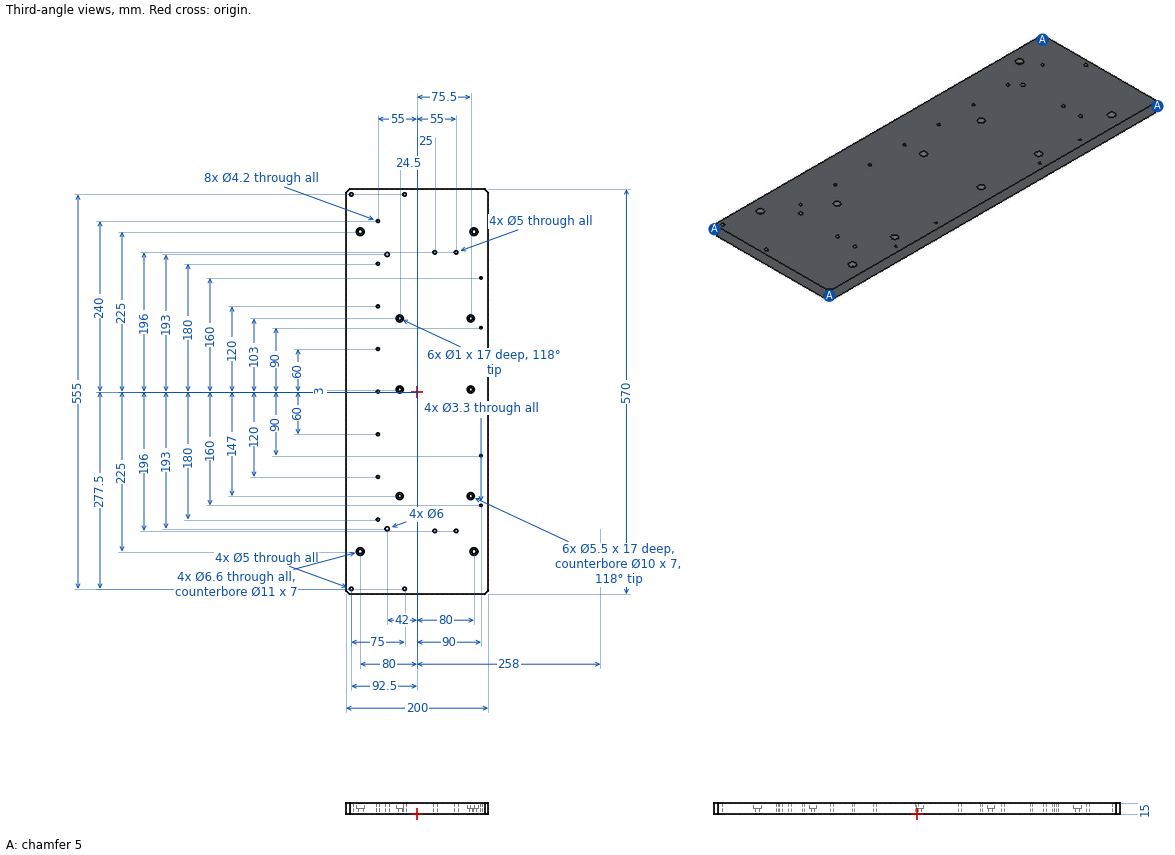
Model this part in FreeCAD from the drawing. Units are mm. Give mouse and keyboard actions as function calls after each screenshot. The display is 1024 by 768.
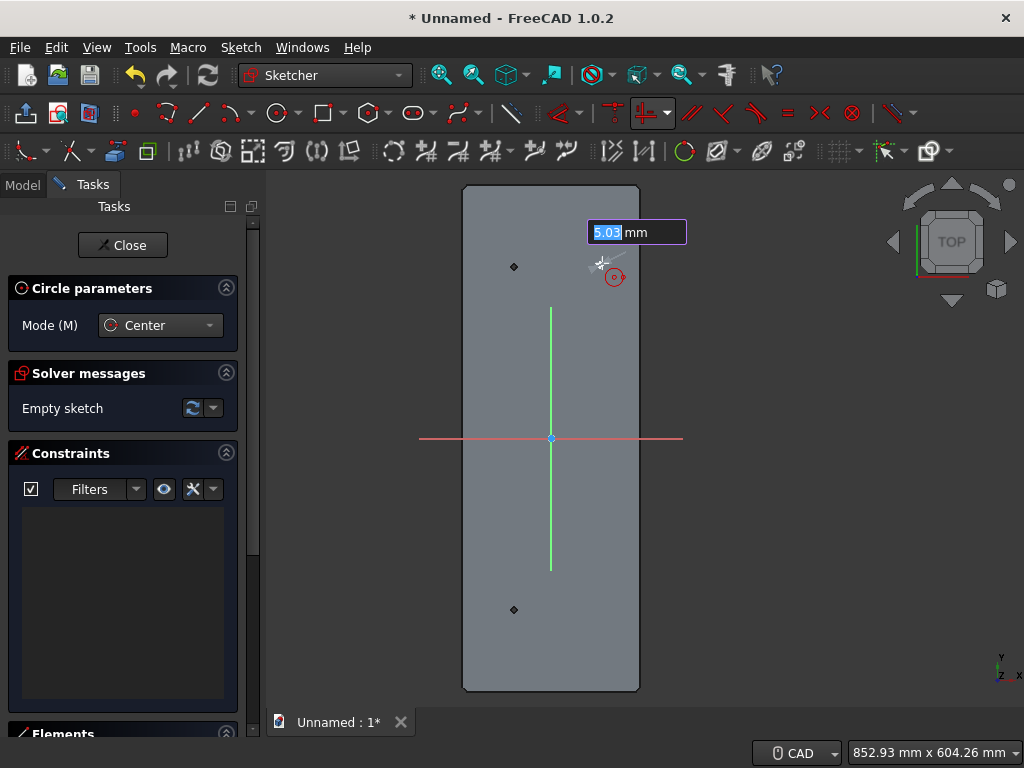
text(5)
key(Return)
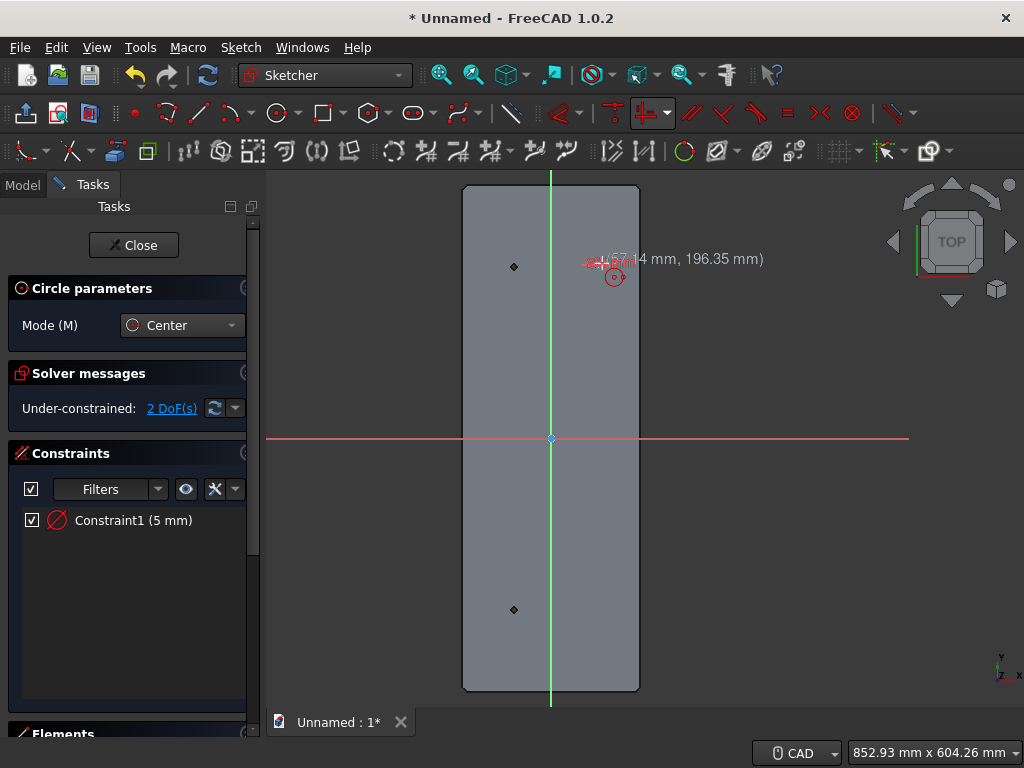
scroll(573, 264, up, 12)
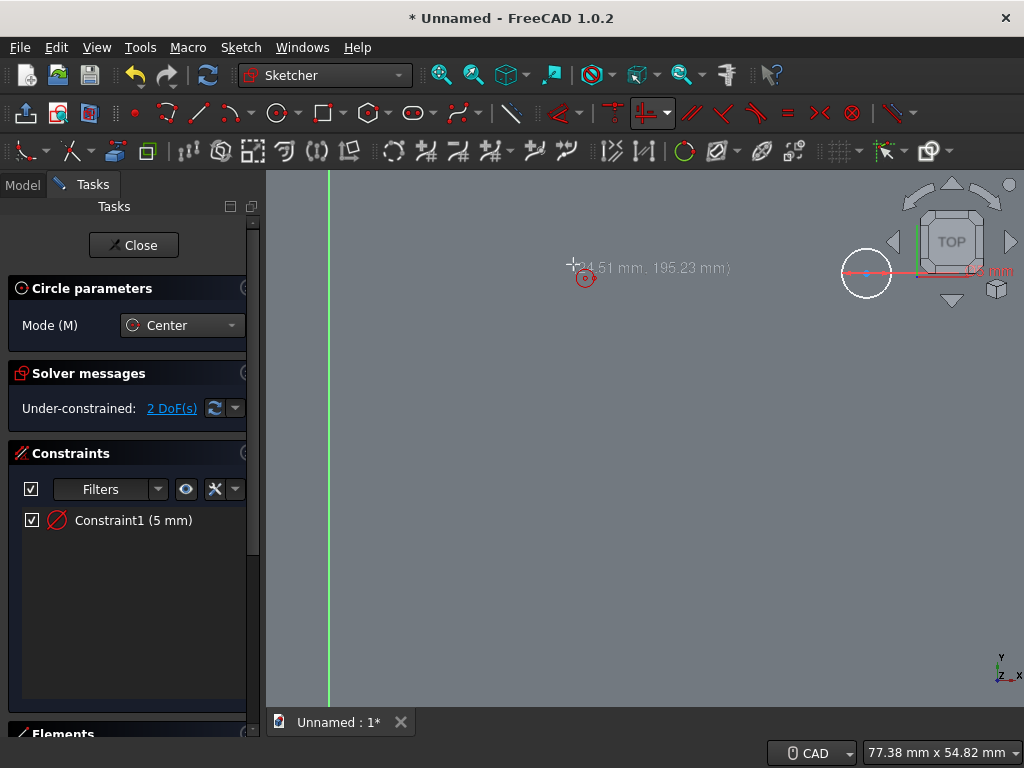
scroll(573, 264, down, 12)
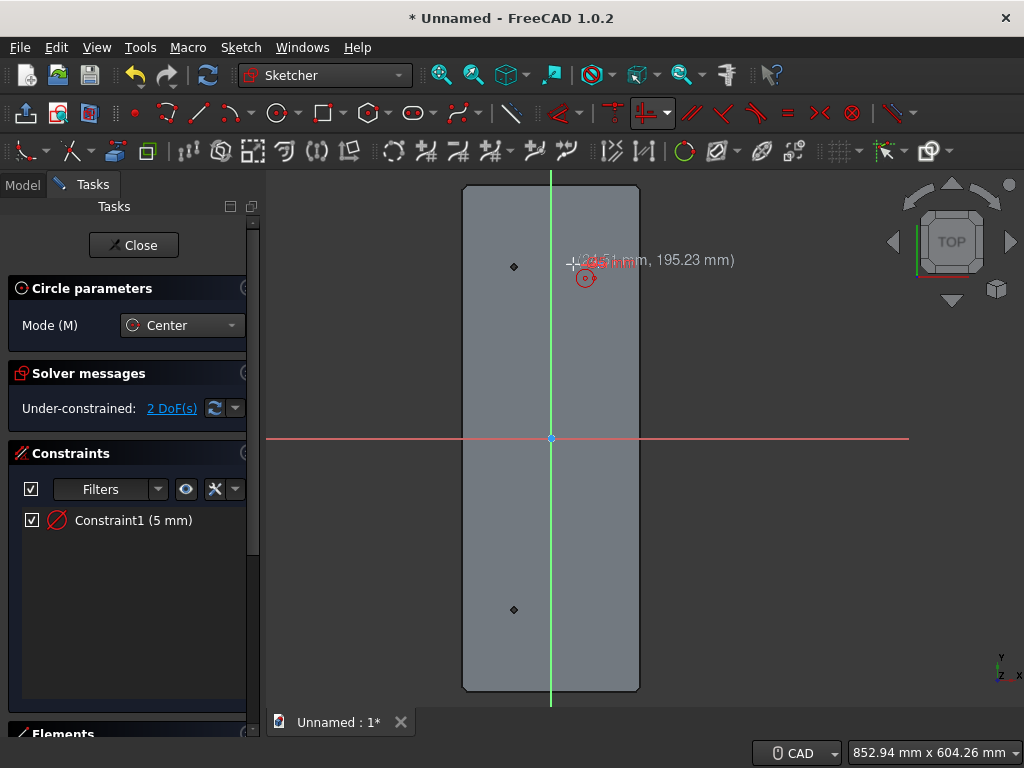
click(573, 264)
move(575, 263)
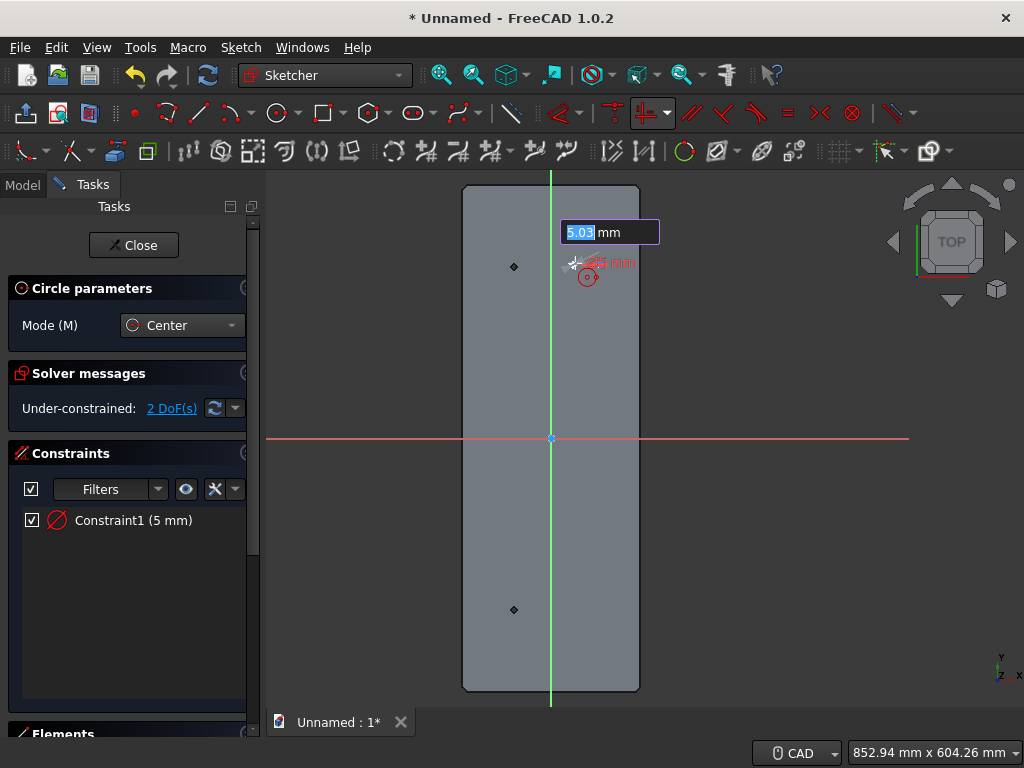
text(5)
key(Return)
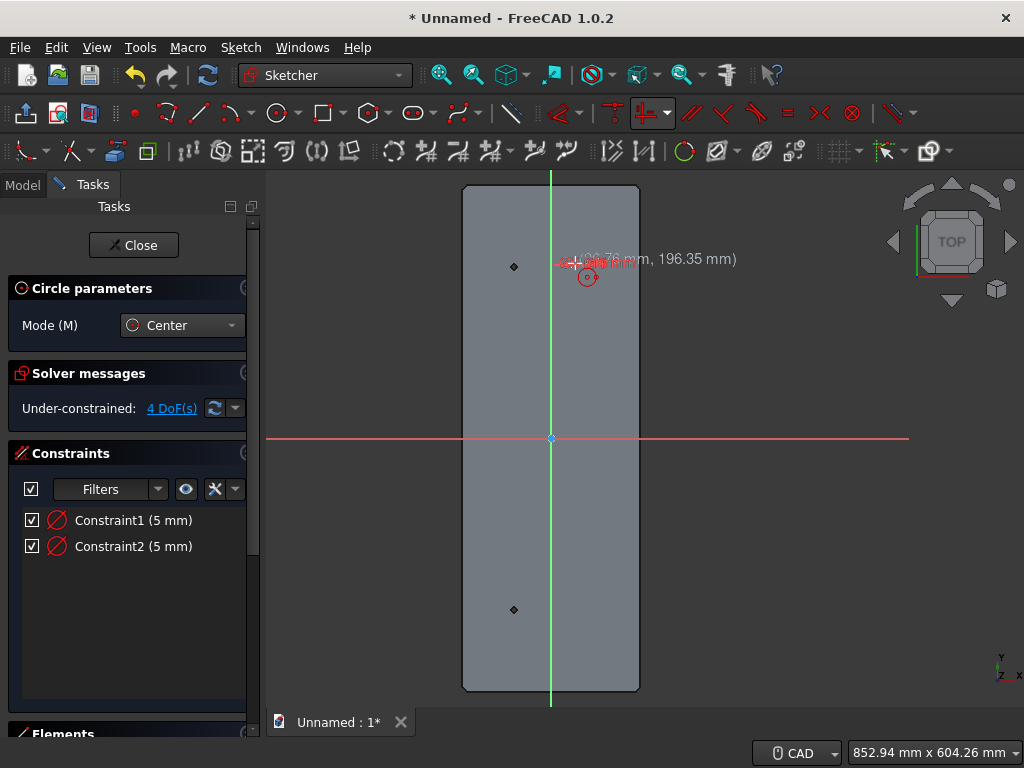
scroll(600, 613, up, 12)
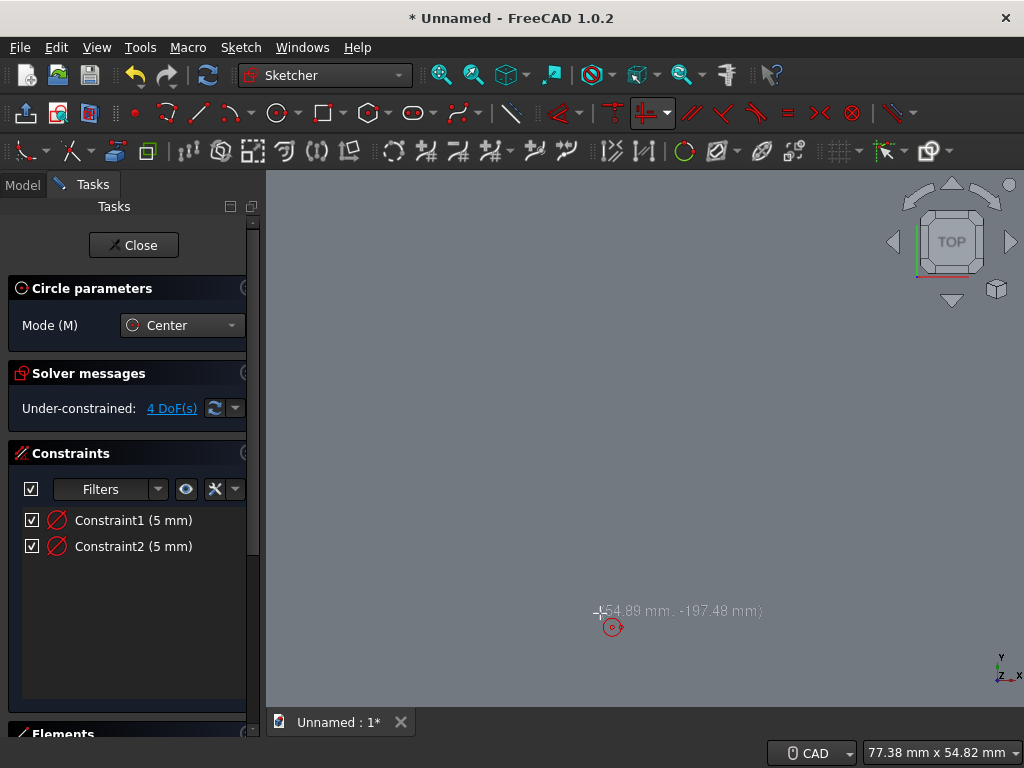
scroll(600, 614, down, 12)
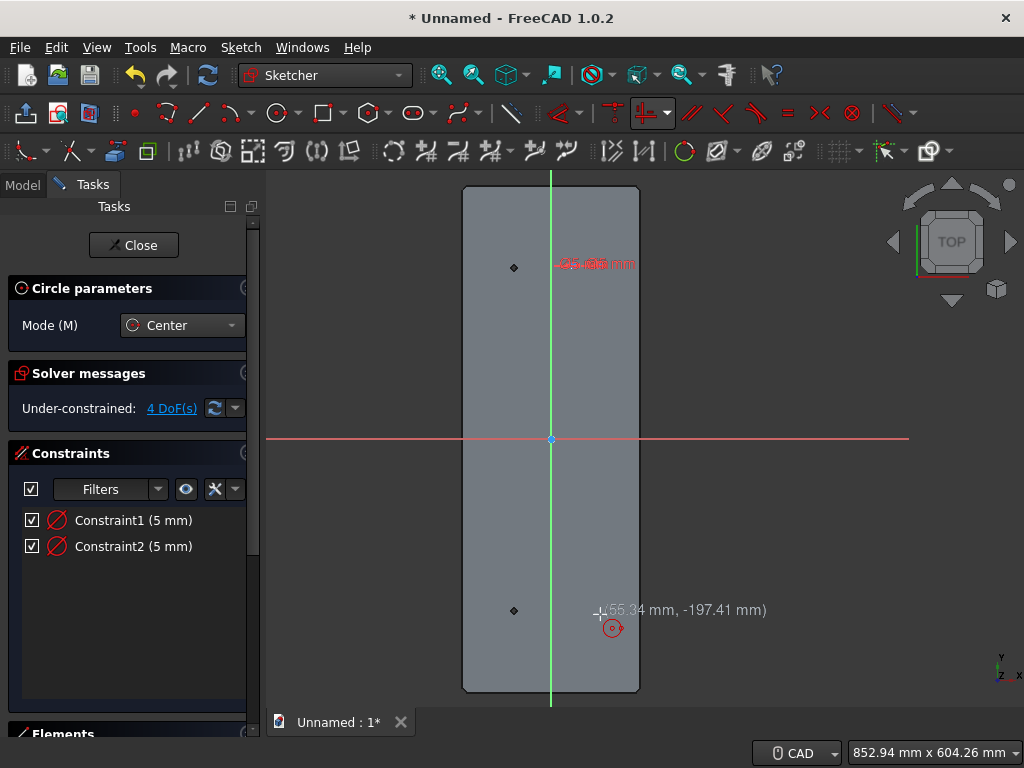
click(600, 614)
move(602, 612)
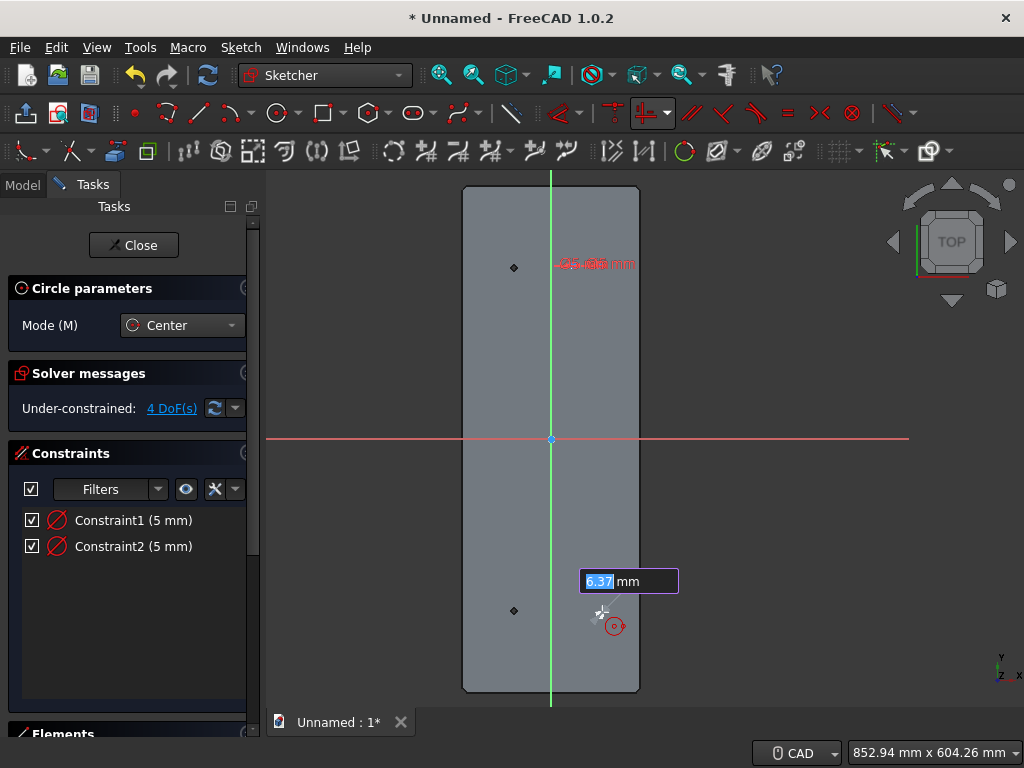
text(5)
key(Return)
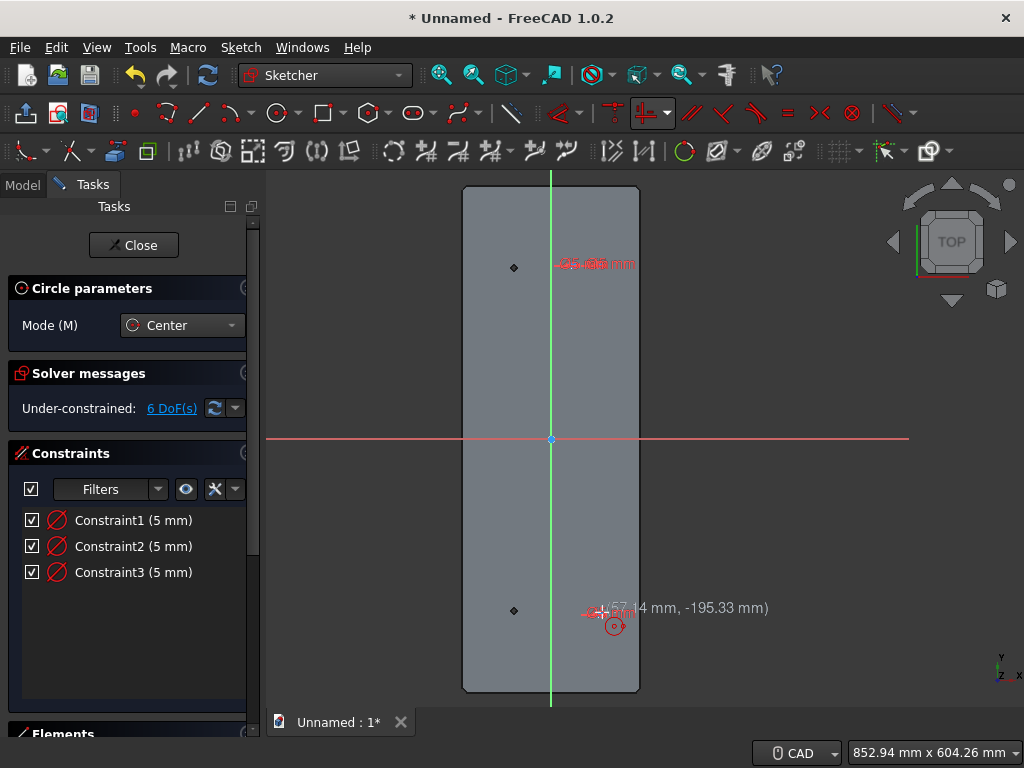
scroll(573, 614, up, 12)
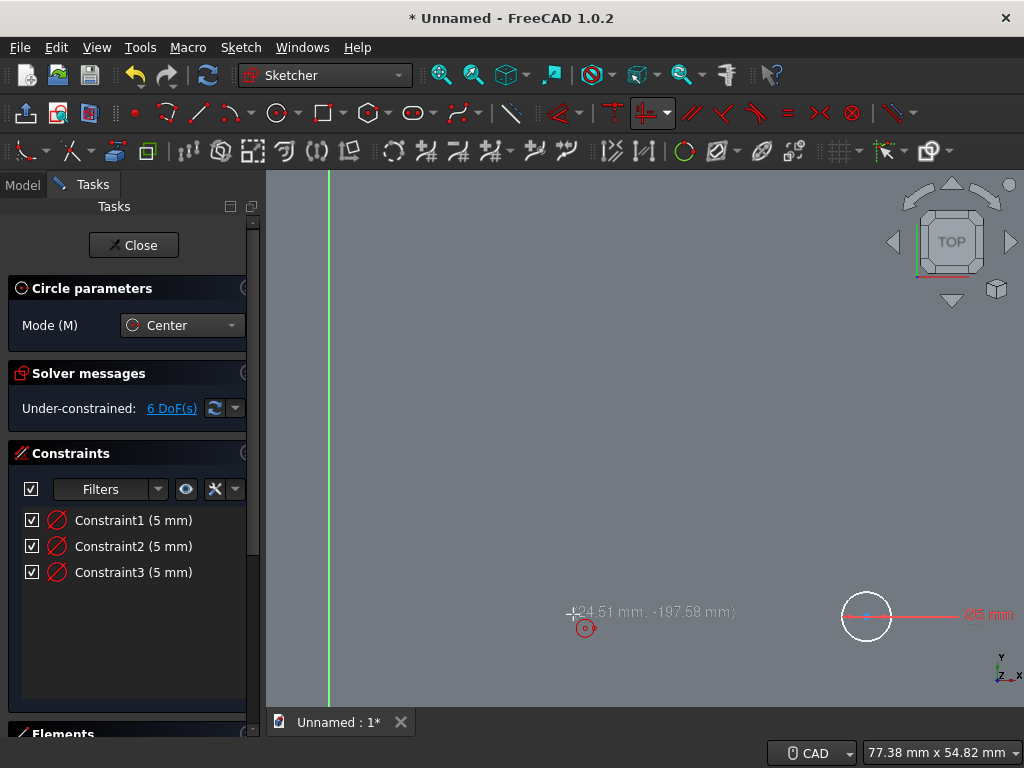
scroll(573, 614, down, 12)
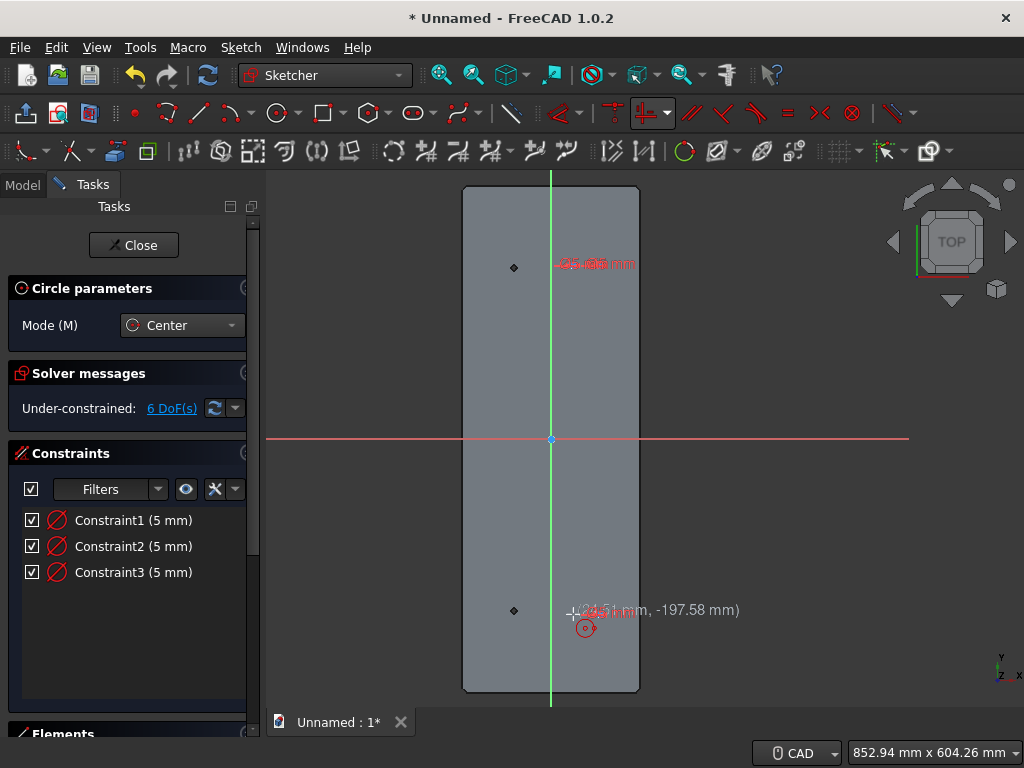
click(573, 614)
move(575, 612)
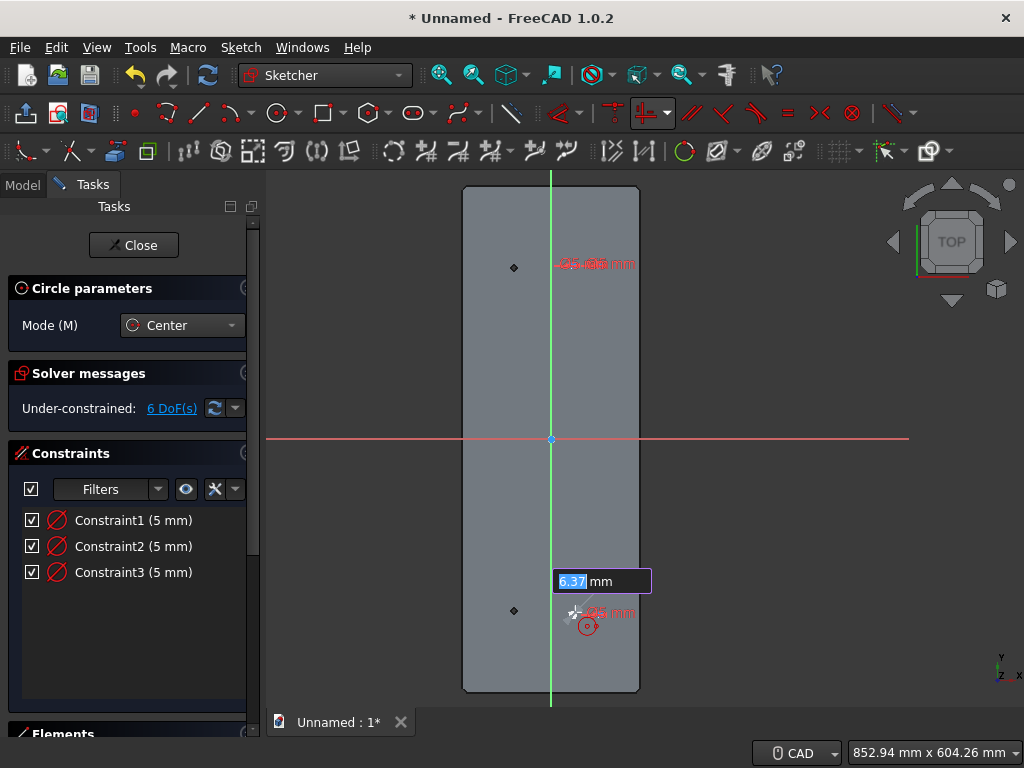
text(5)
key(Return)
key(Escape)